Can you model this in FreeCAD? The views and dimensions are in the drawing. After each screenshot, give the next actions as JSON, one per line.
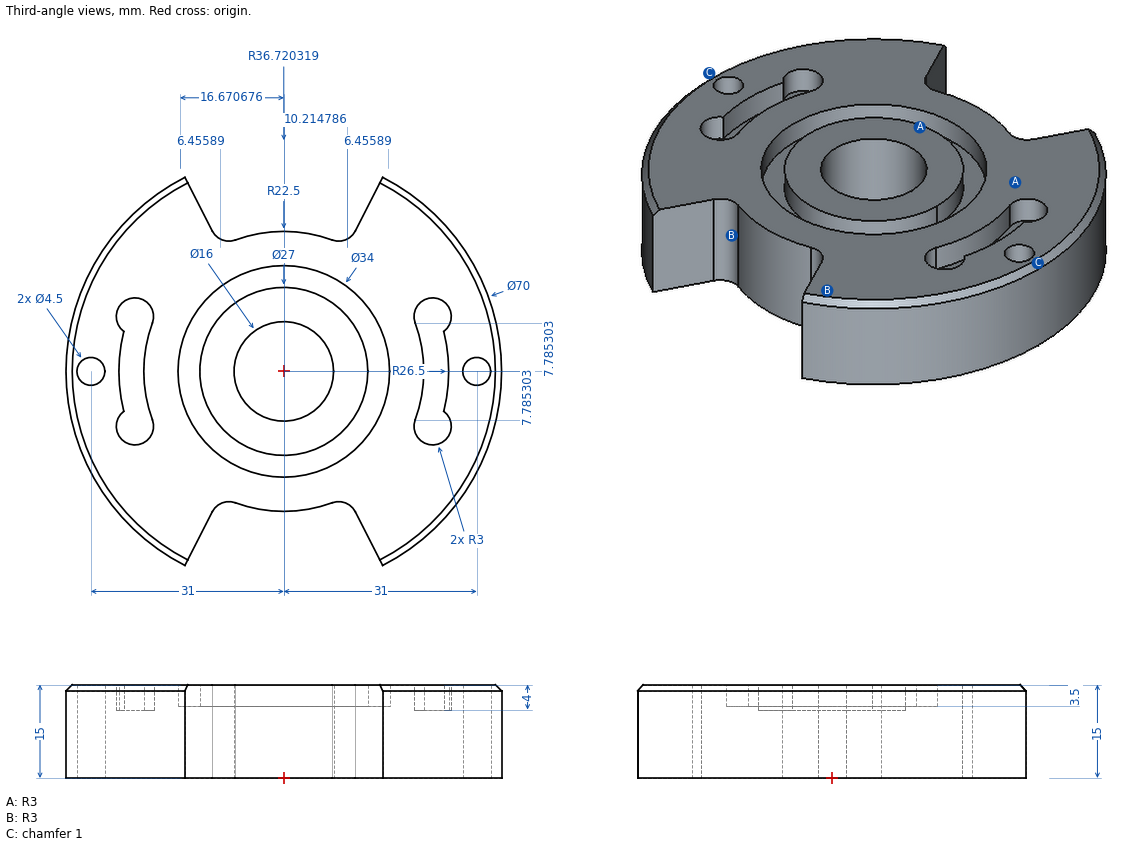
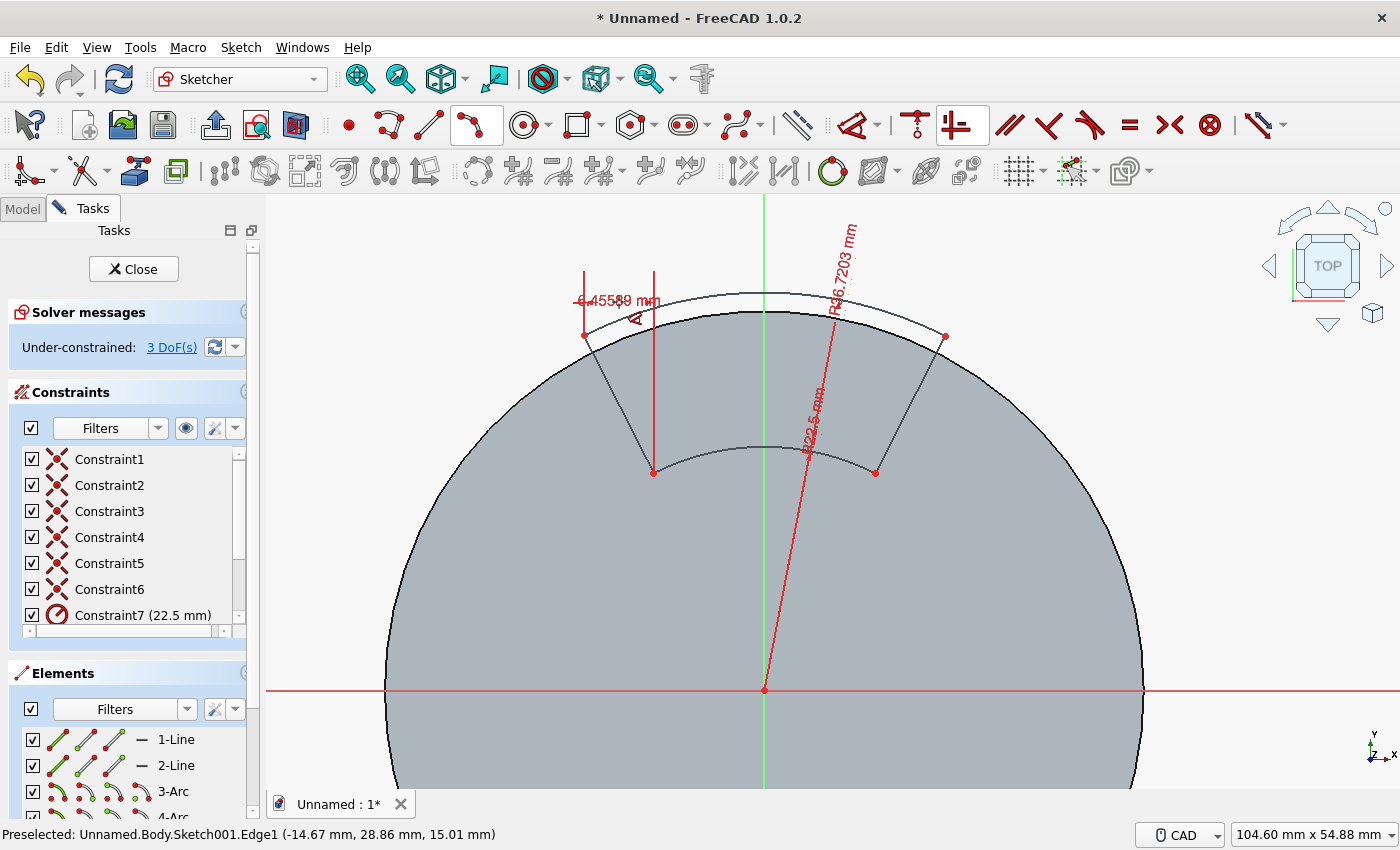
{"action": "left_click", "coordinate": [896, 432]}
{"action": "left_click", "coordinate": [910, 302]}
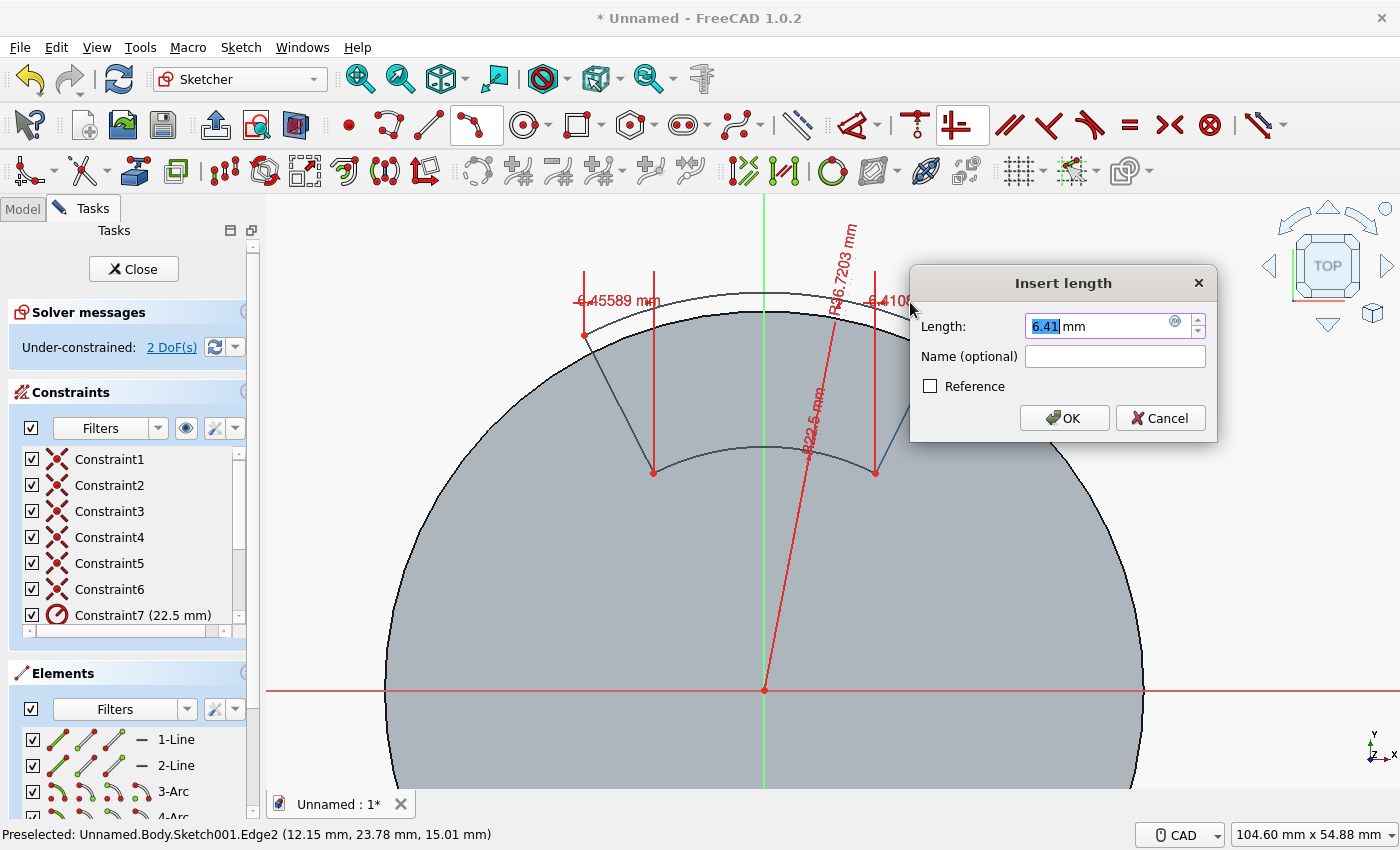
{"action": "type", "text": "6.45589"}
{"action": "key", "text": "Return"}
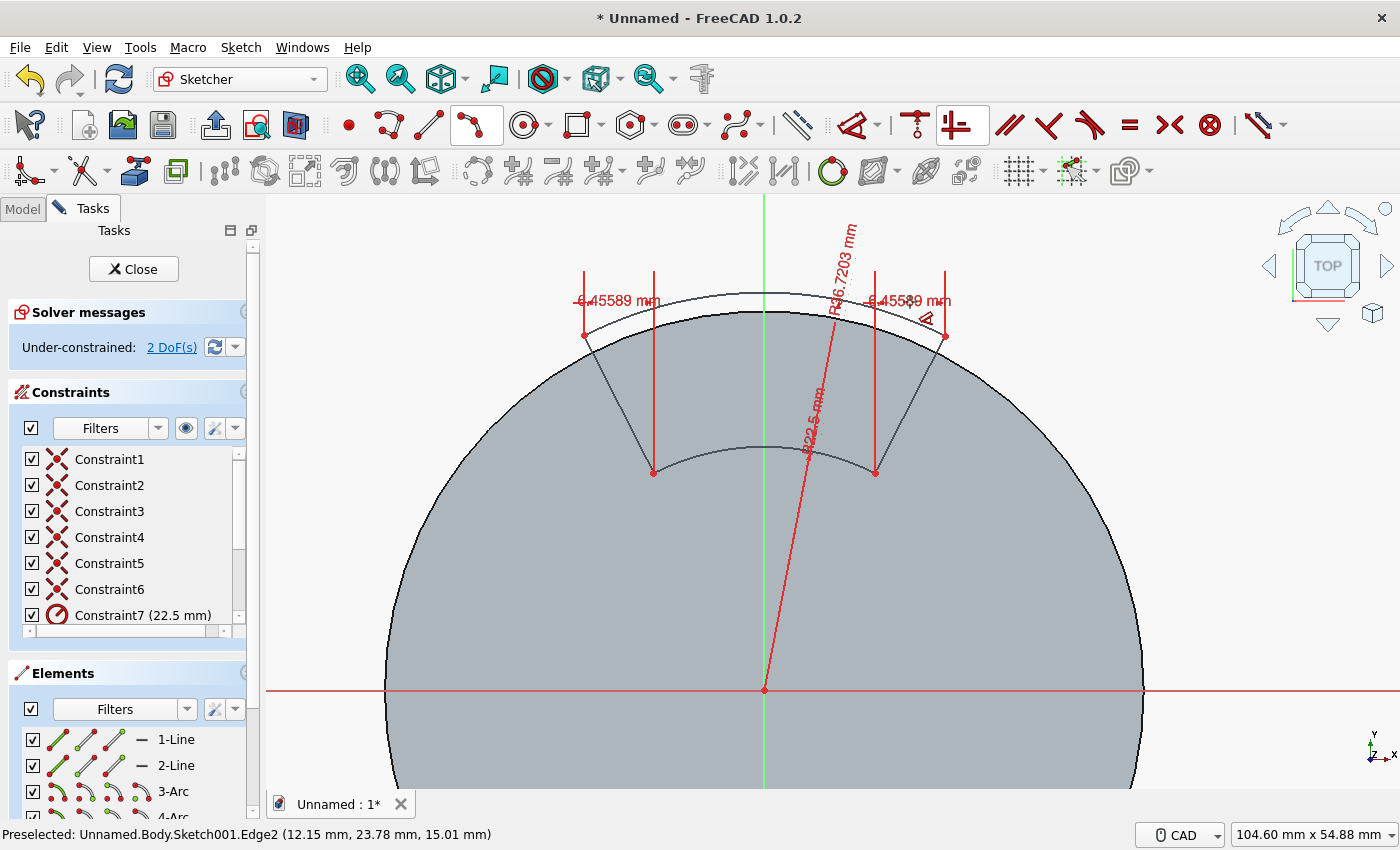
{"action": "left_click", "coordinate": [584, 336]}
{"action": "left_click", "coordinate": [674, 725]}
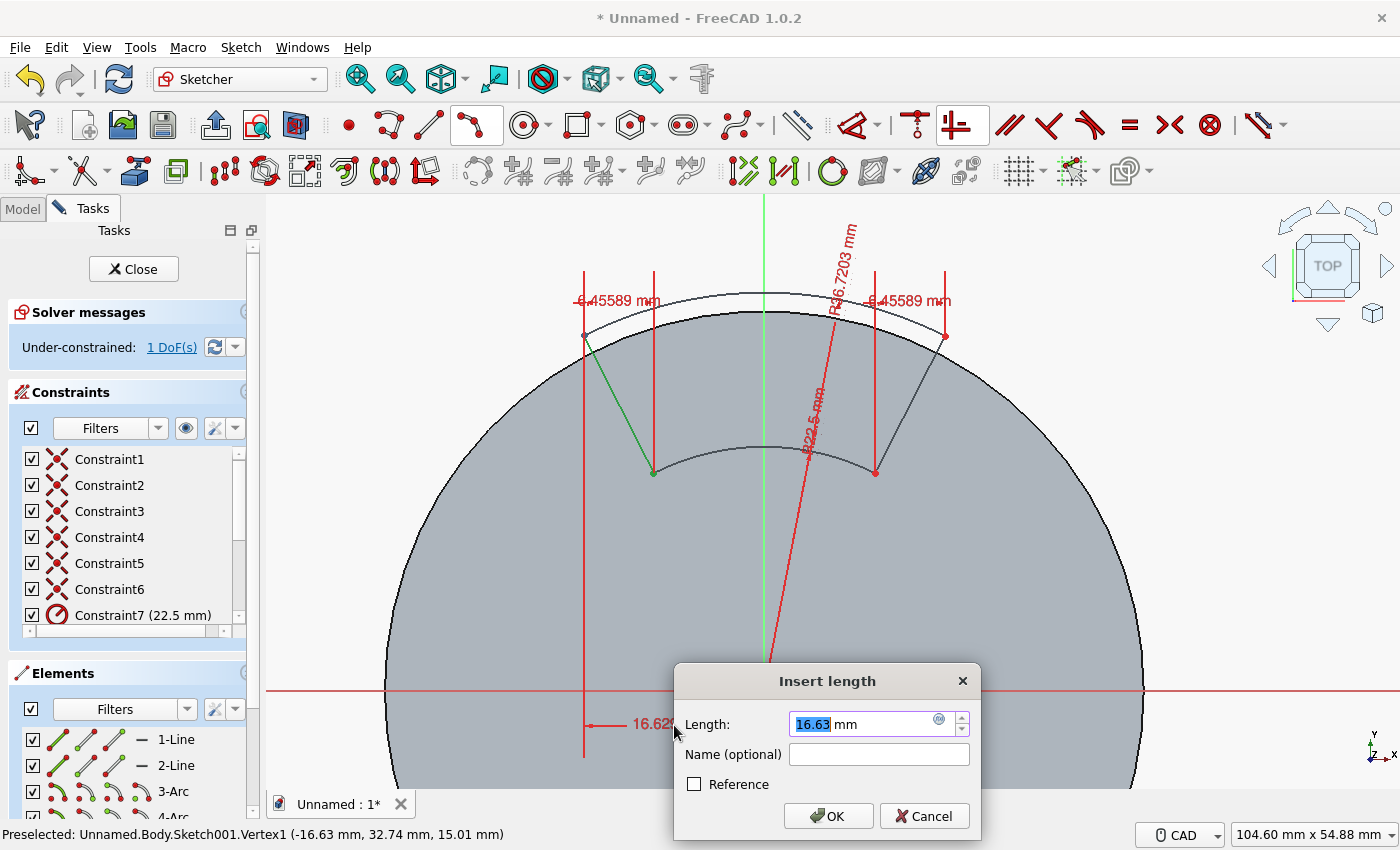
{"action": "type", "text": "16.670676"}
{"action": "key", "text": "Return"}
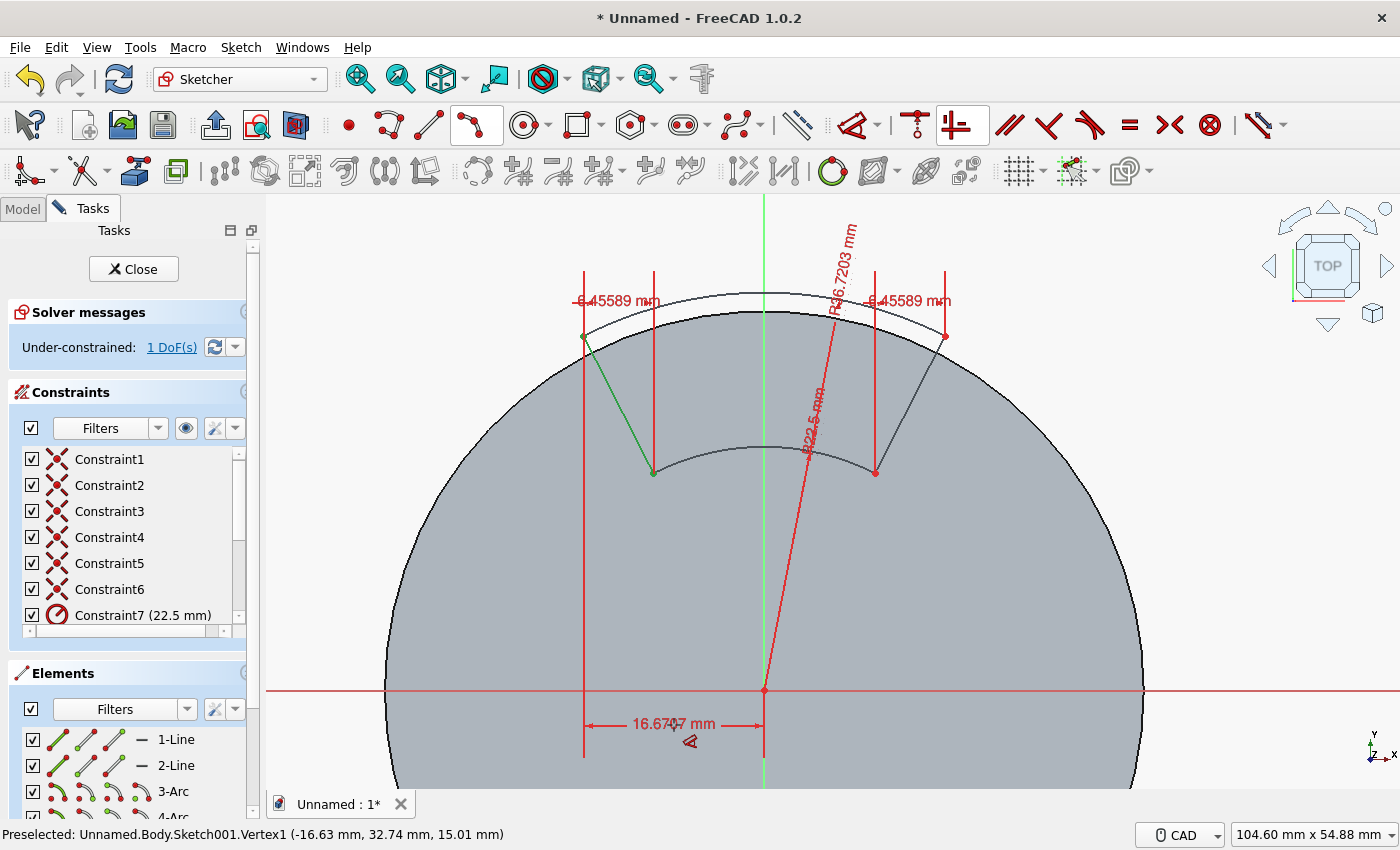
{"action": "left_click", "coordinate": [875, 473]}
{"action": "left_click", "coordinate": [820, 725]}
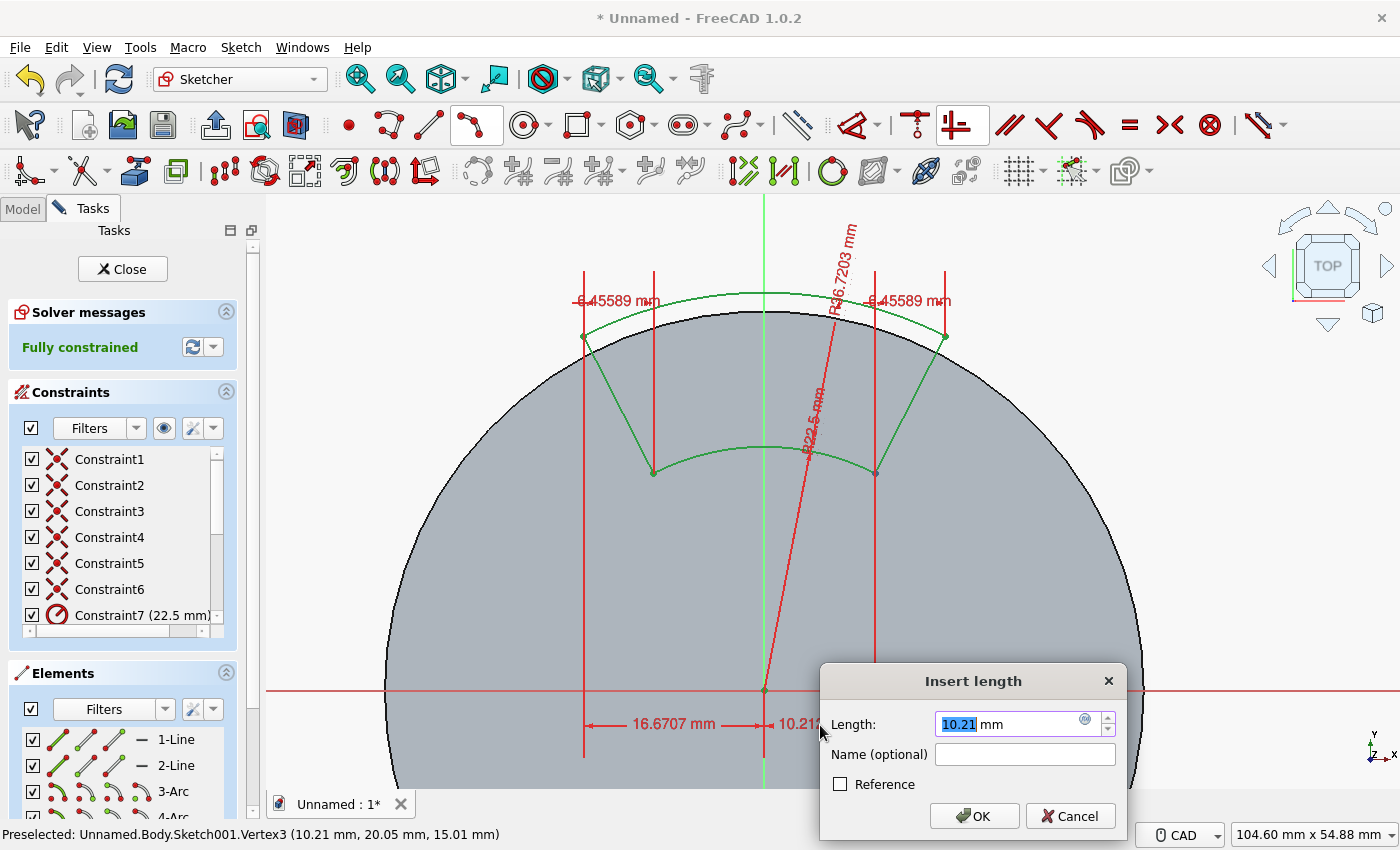
{"action": "type", "text": "10.214786"}
{"action": "key", "text": "Return"}
{"action": "key", "text": "Escape"}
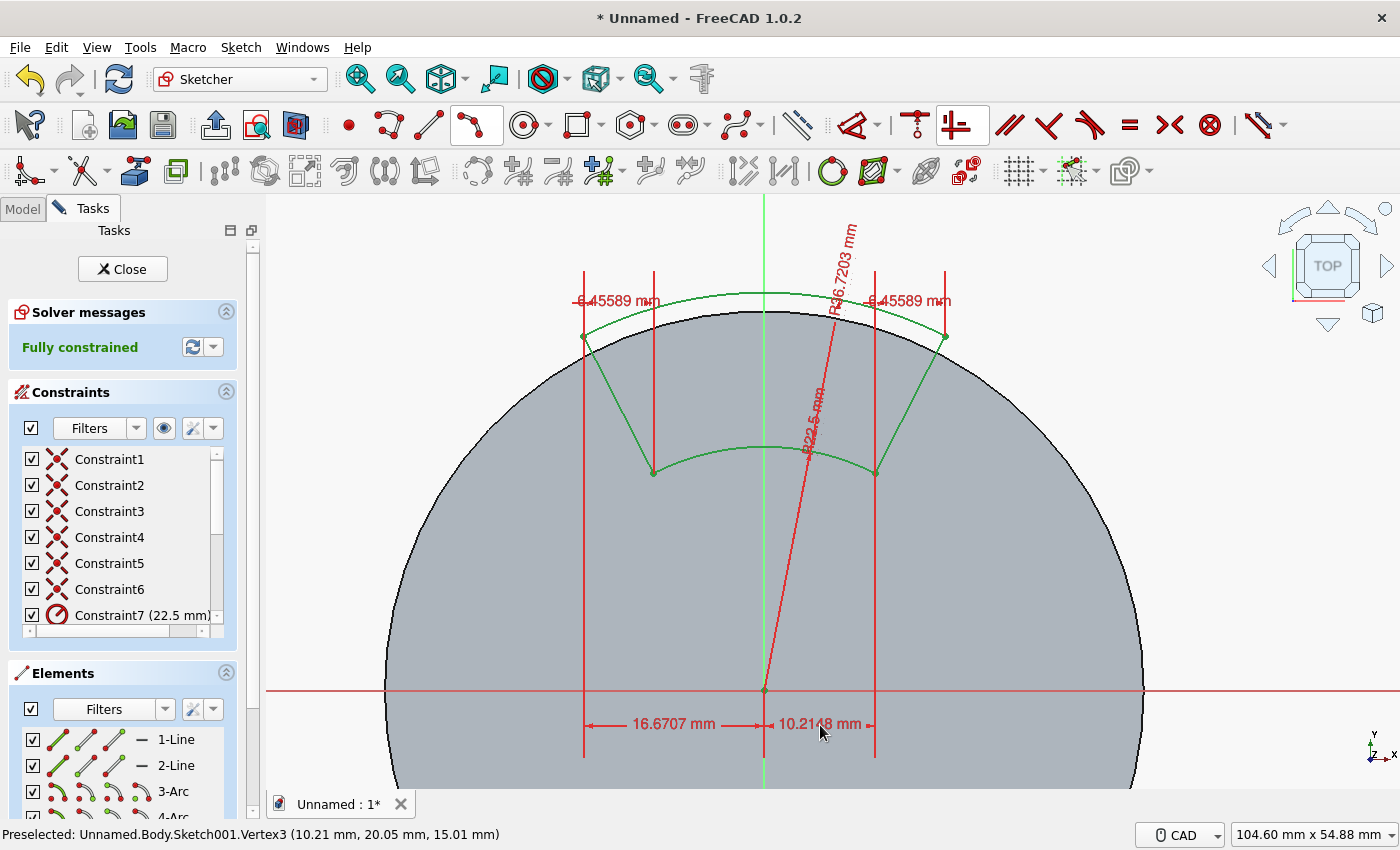
{"action": "left_click", "coordinate": [123, 269]}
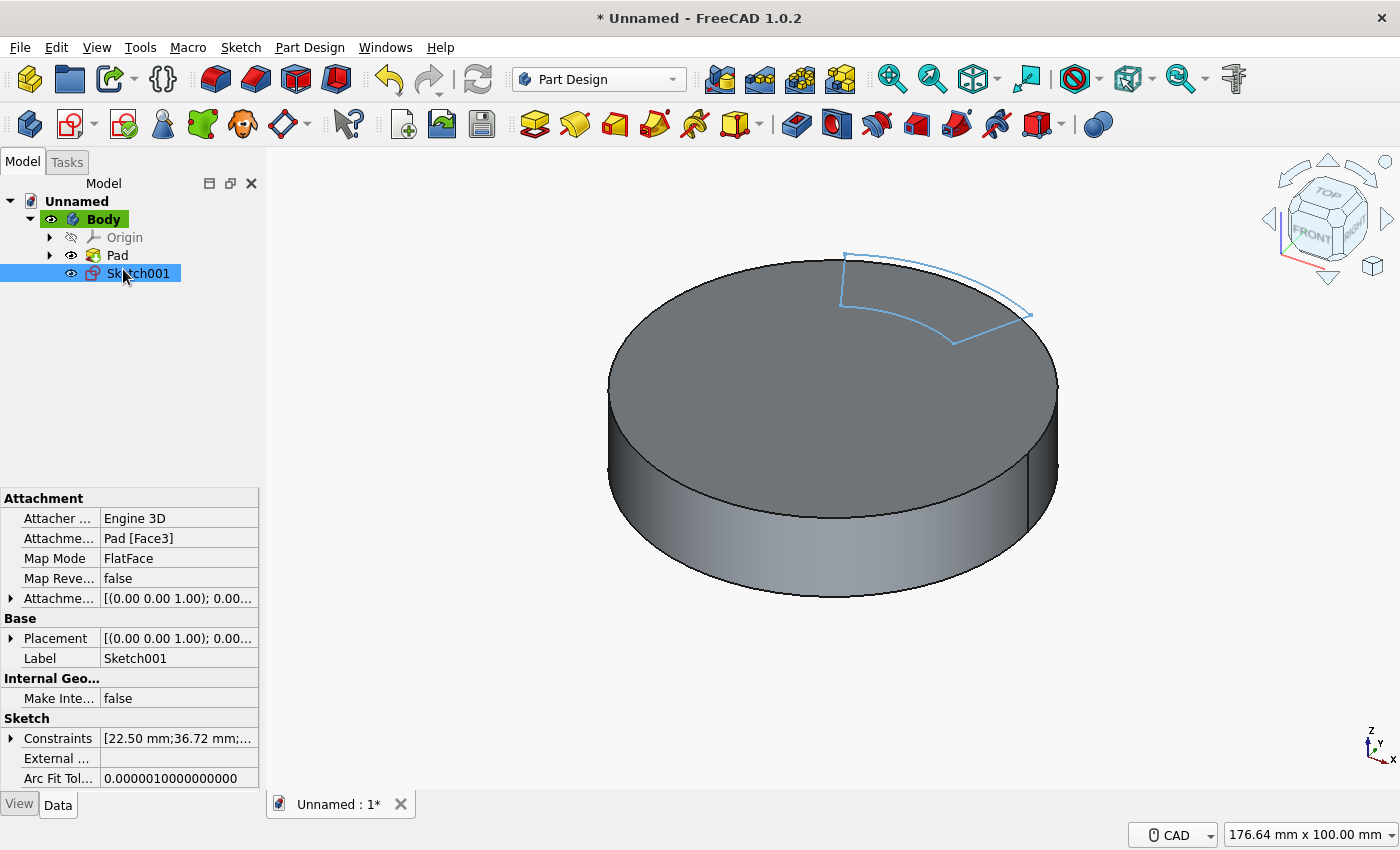
{"action": "left_click", "coordinate": [798, 124]}